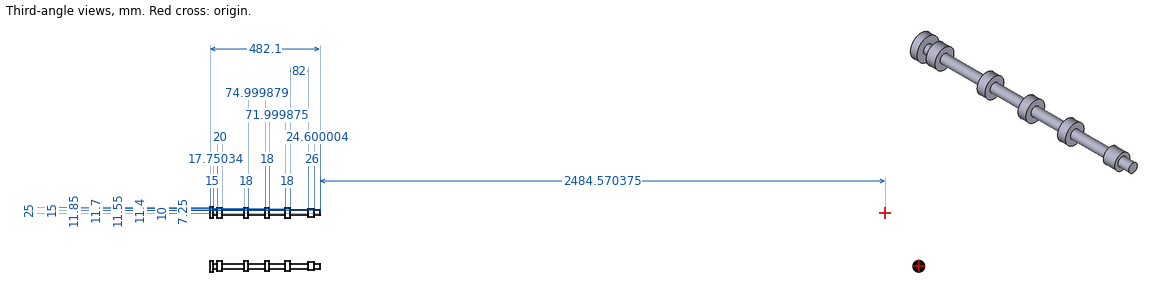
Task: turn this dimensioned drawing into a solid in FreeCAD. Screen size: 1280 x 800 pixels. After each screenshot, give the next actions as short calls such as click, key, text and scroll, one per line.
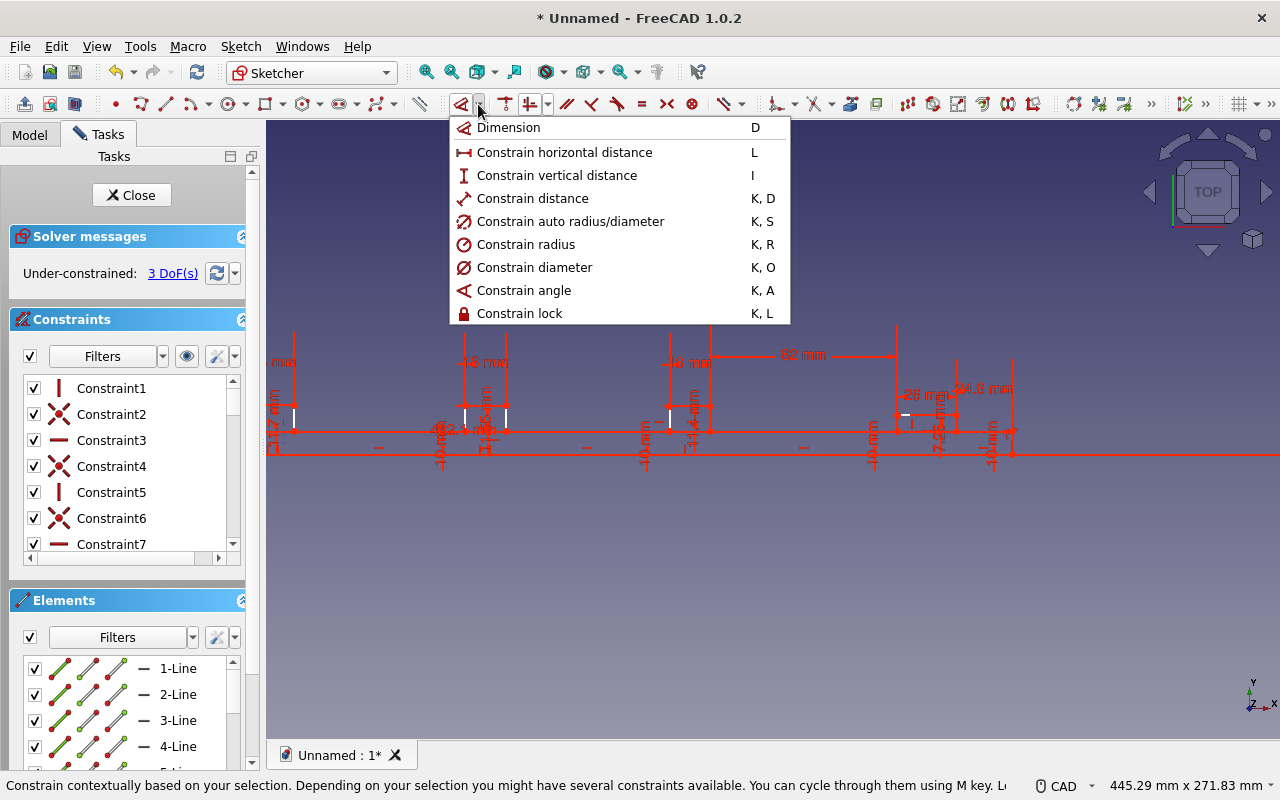
click(620, 152)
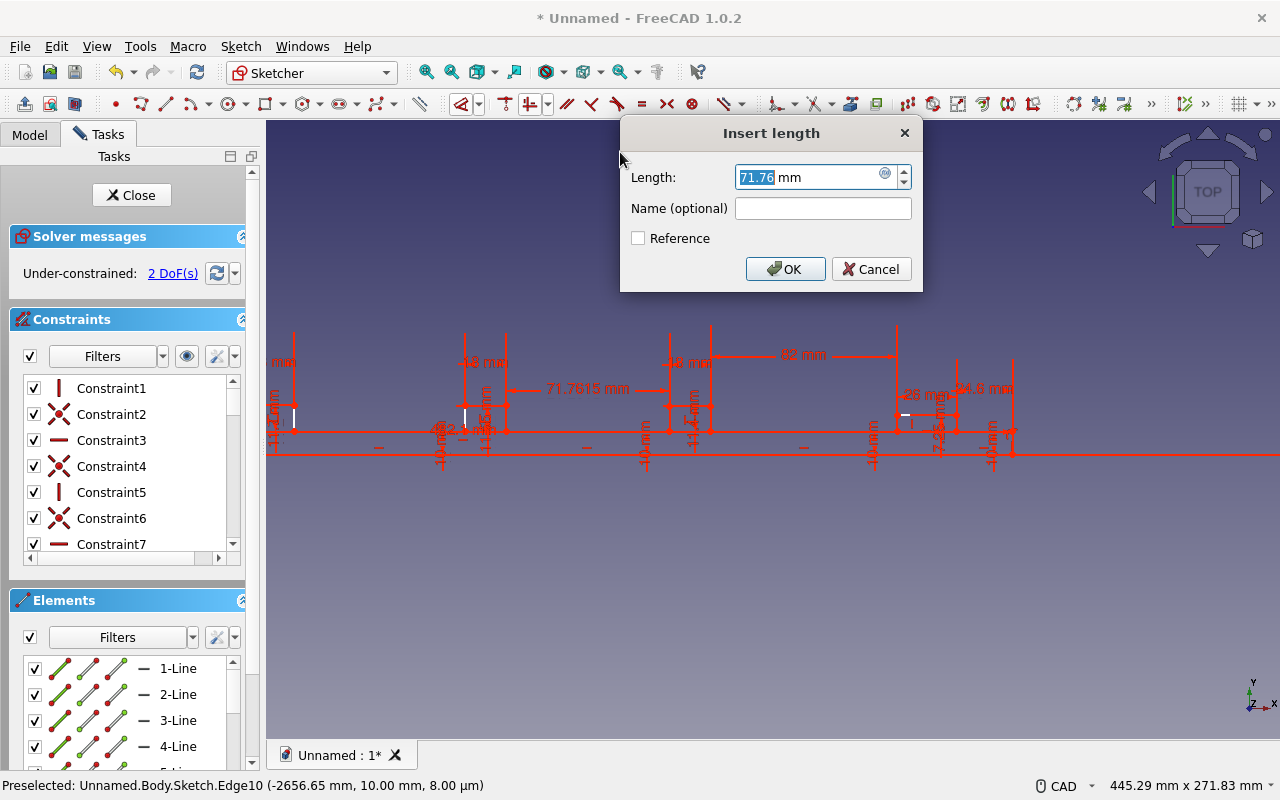
text(71.999875)
key(Return)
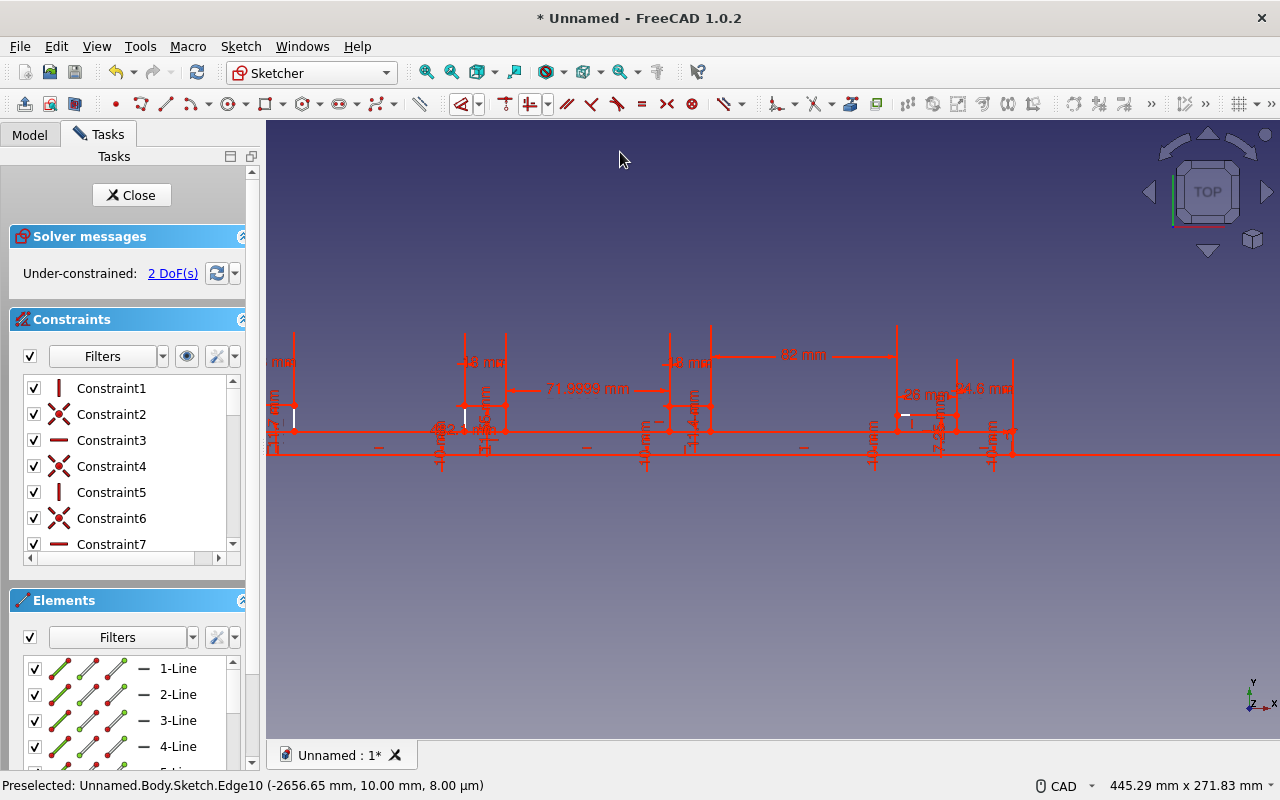
click(414, 432)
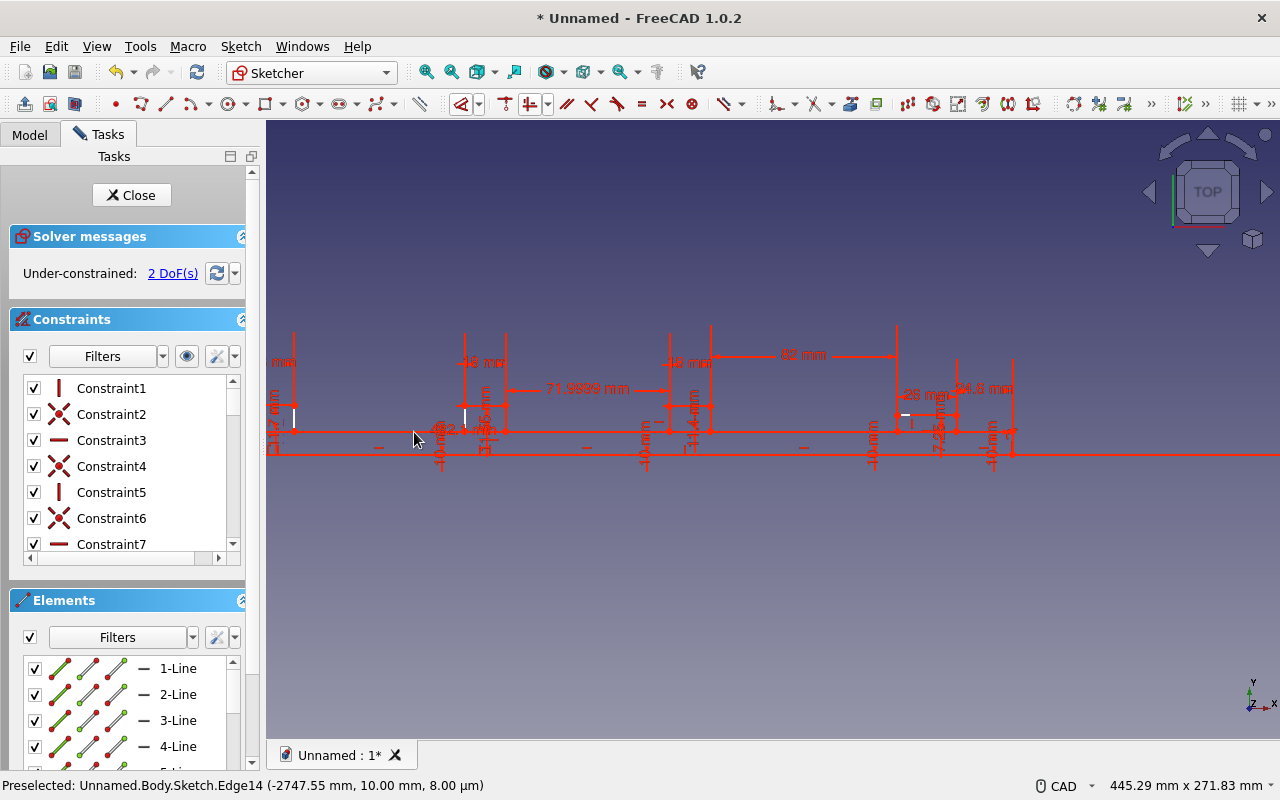
key(l)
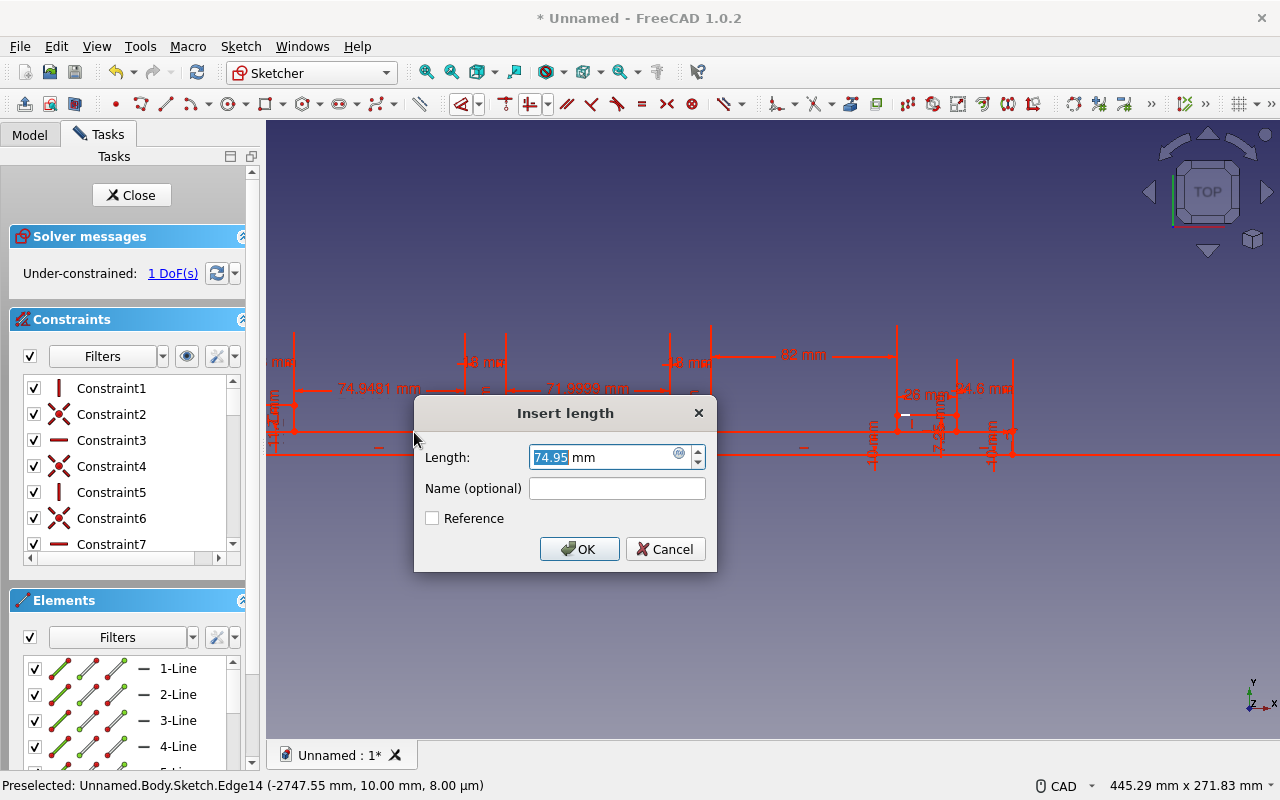
text(74.999879)
key(Return)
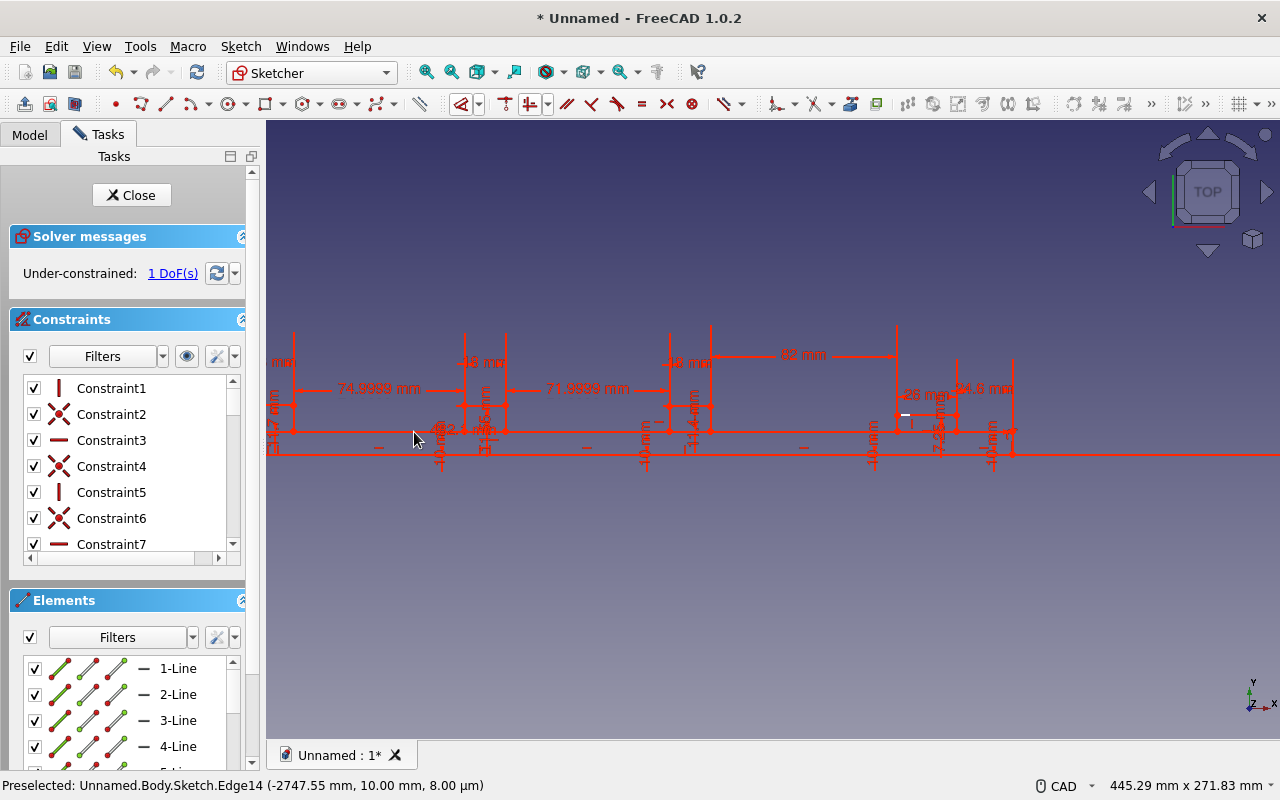
click(1013, 455)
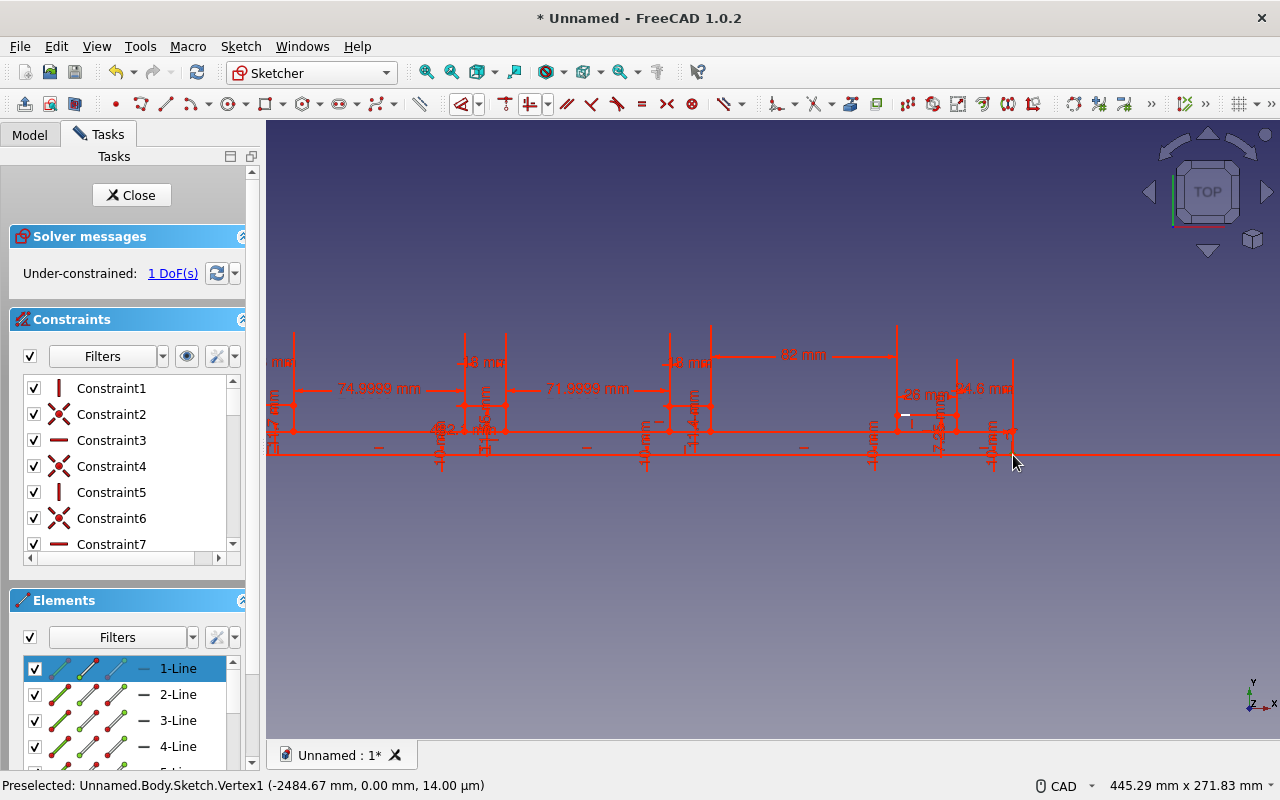
click(478, 104)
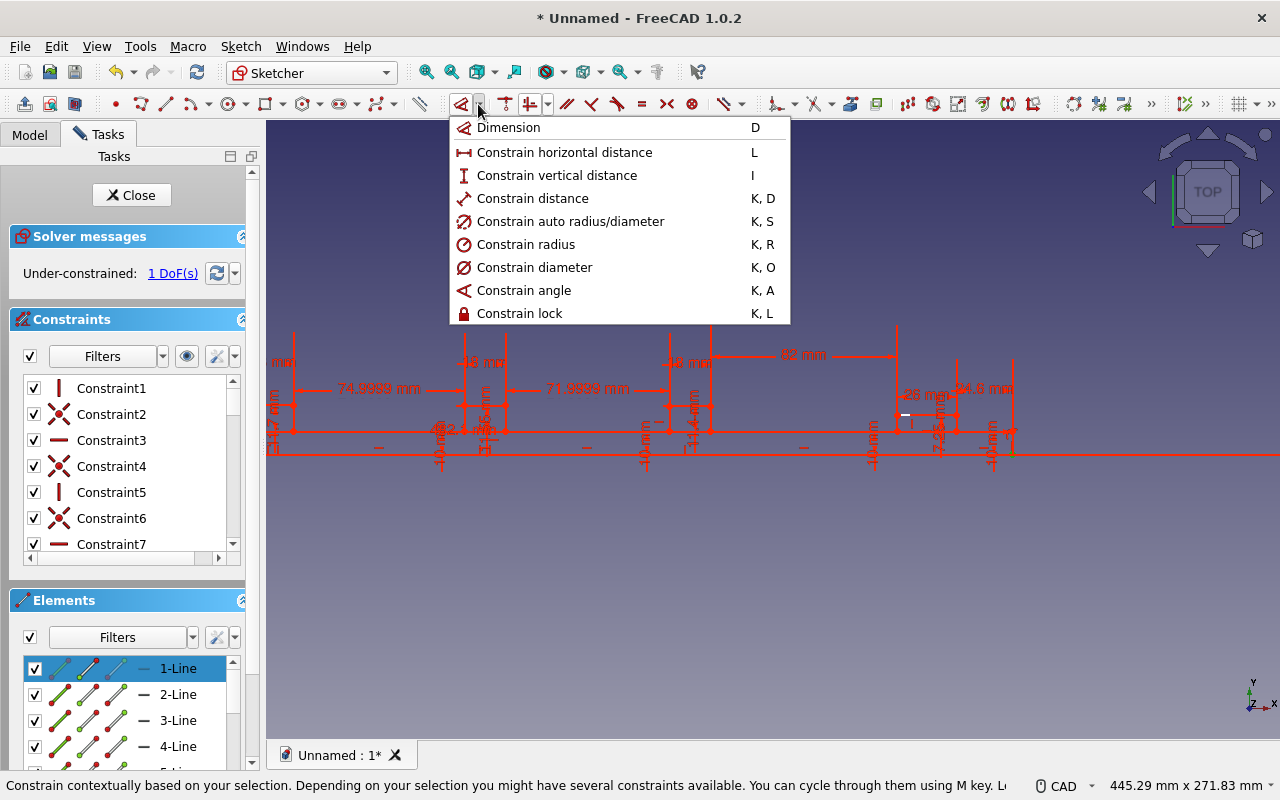
click(620, 152)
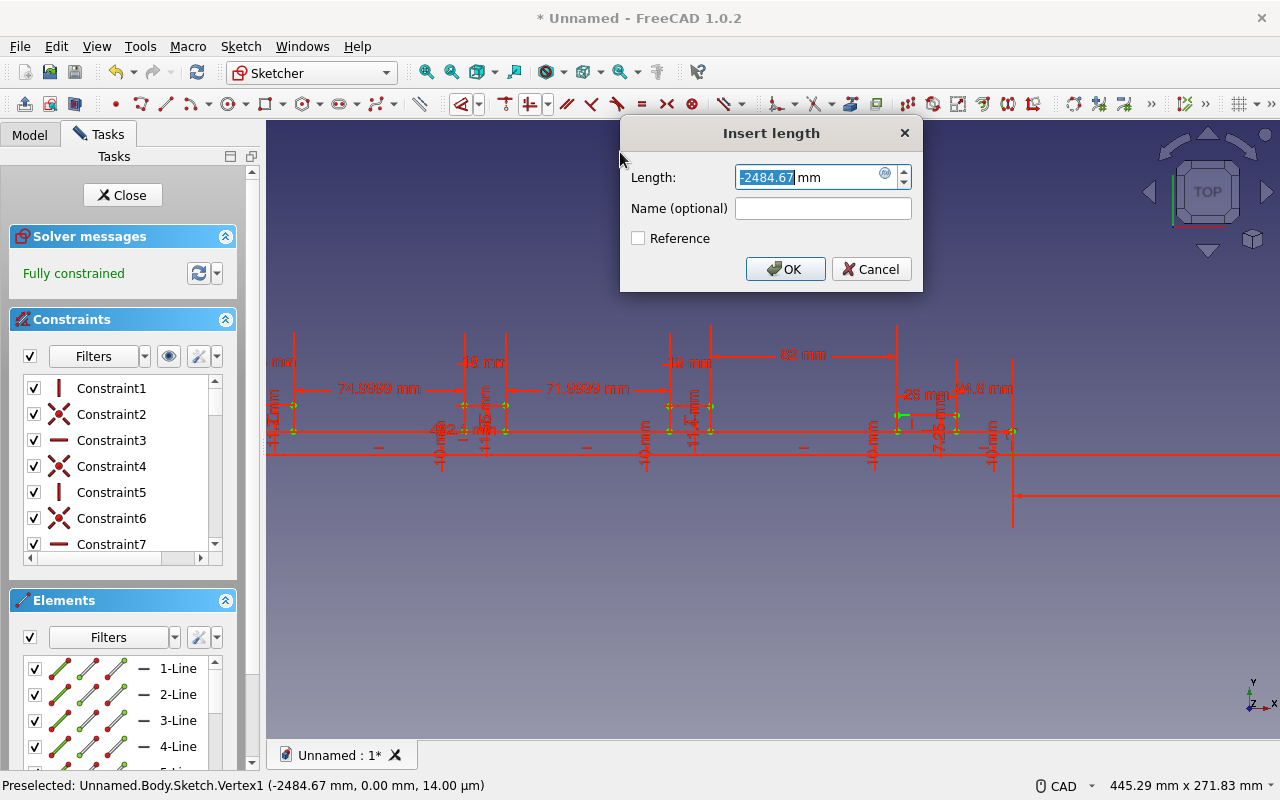
text(-2484.570375)
key(Return)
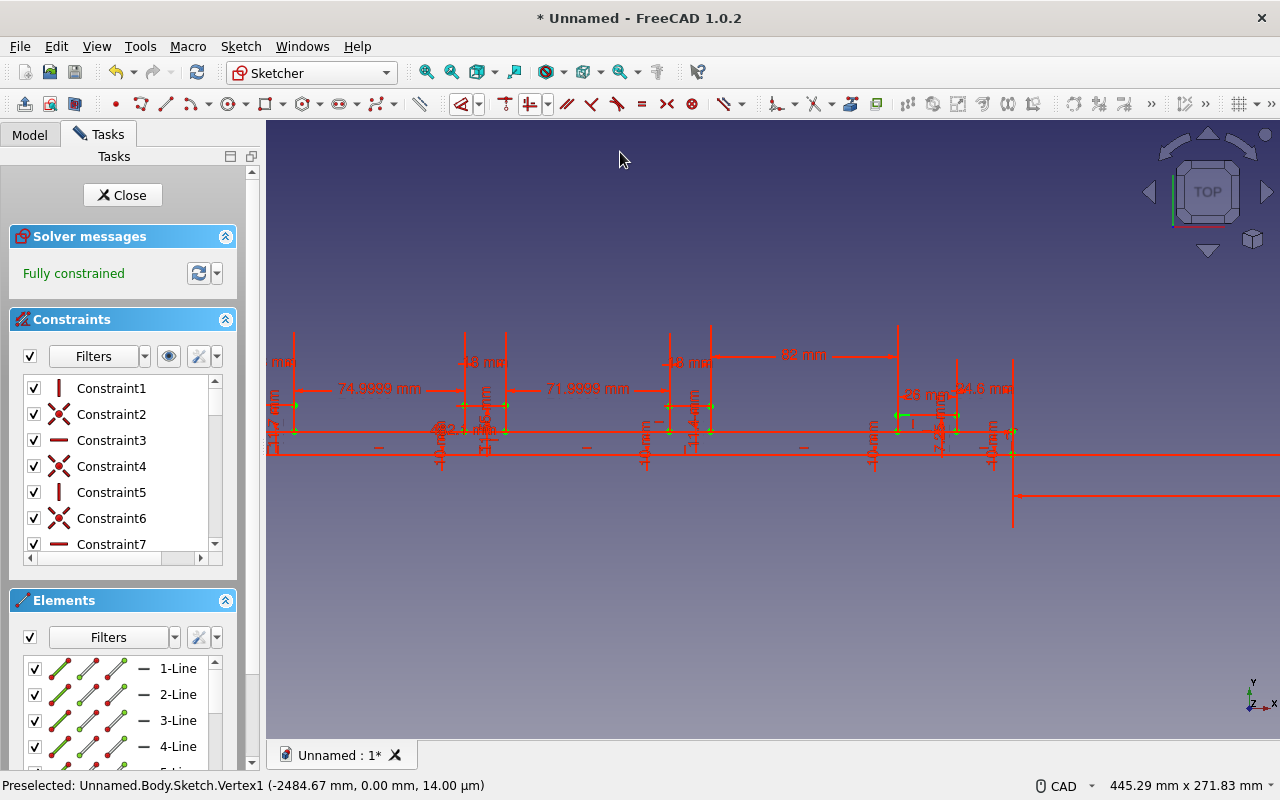
click(123, 195)